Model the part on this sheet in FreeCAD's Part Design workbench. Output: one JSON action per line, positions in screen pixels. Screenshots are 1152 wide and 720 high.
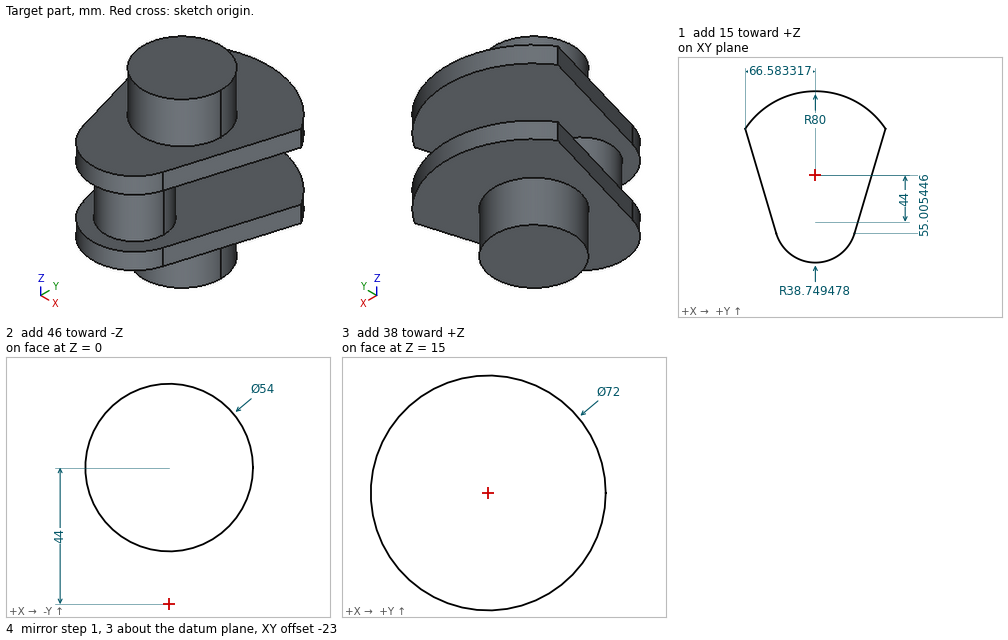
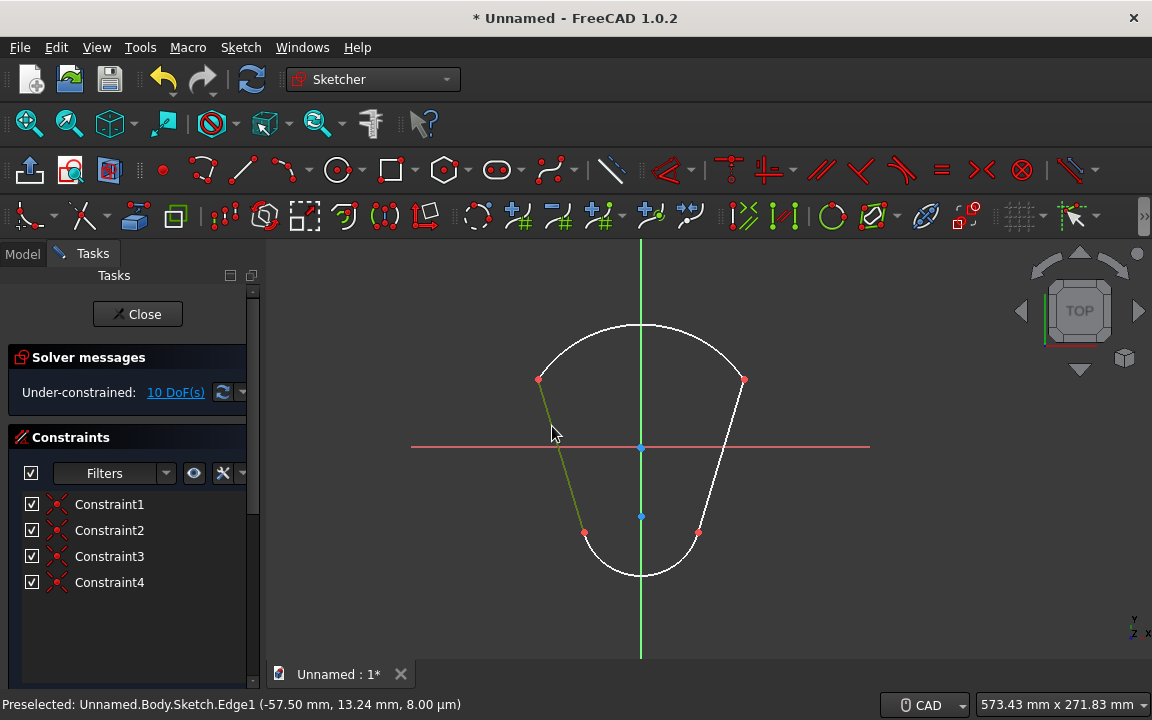
{"action": "left_click", "coordinate": [612, 568]}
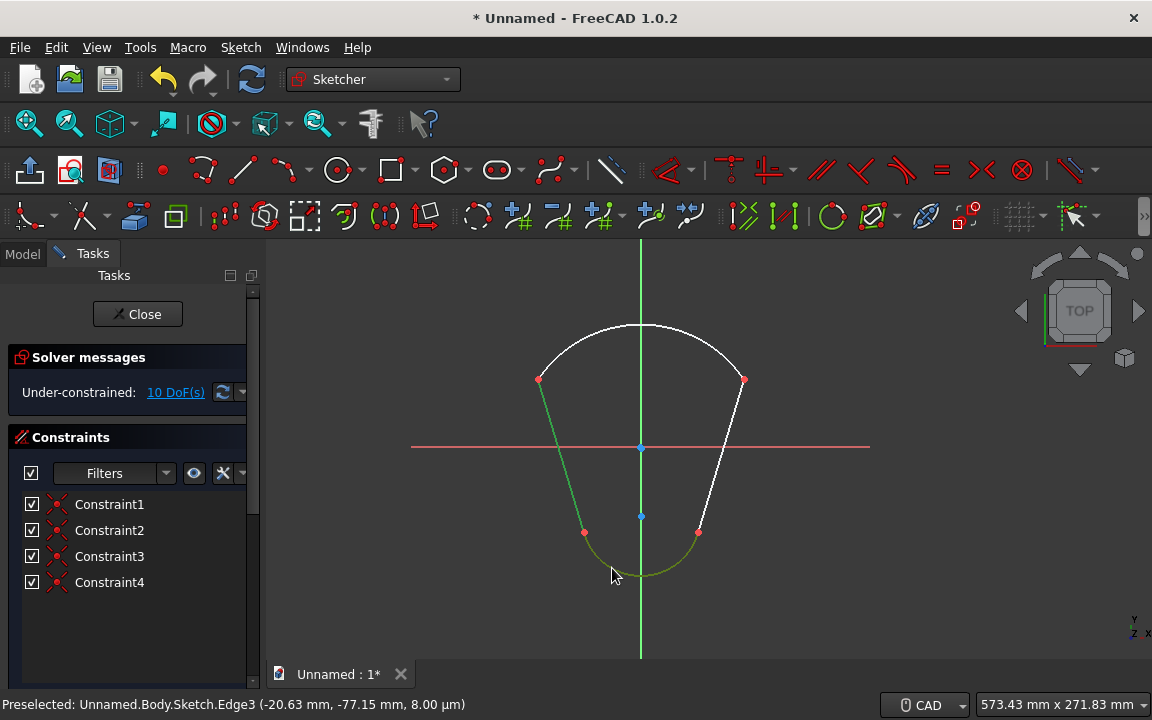
{"action": "key", "text": "t"}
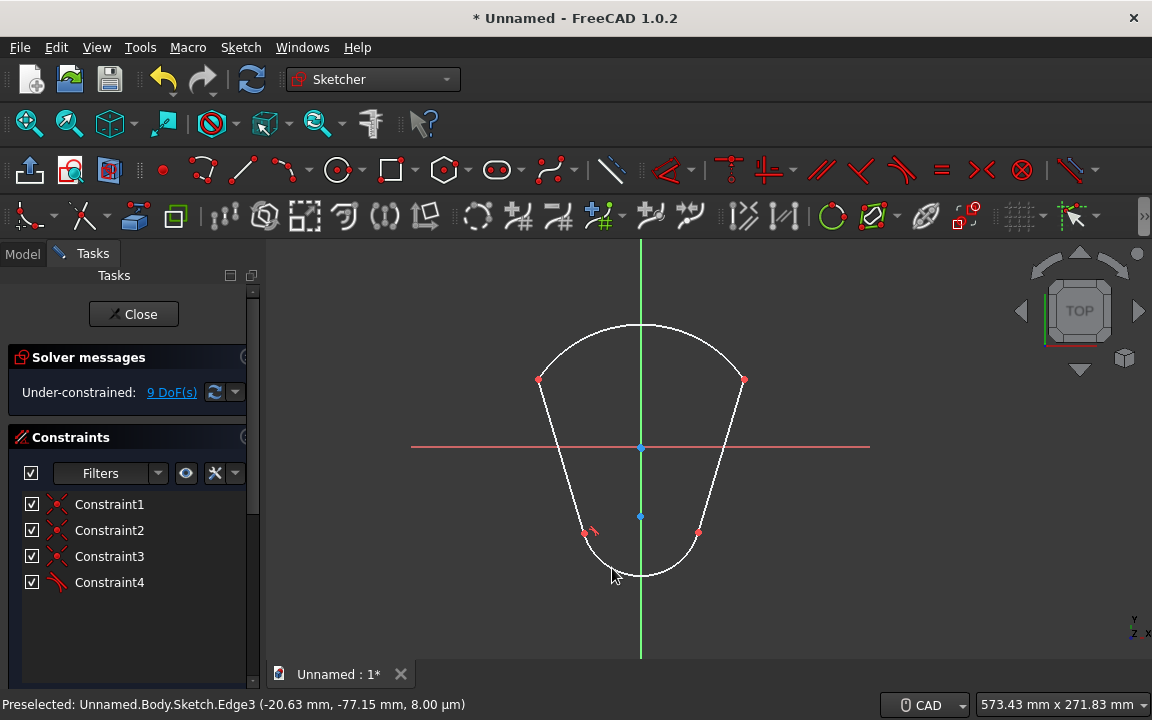
{"action": "left_click", "coordinate": [712, 487]}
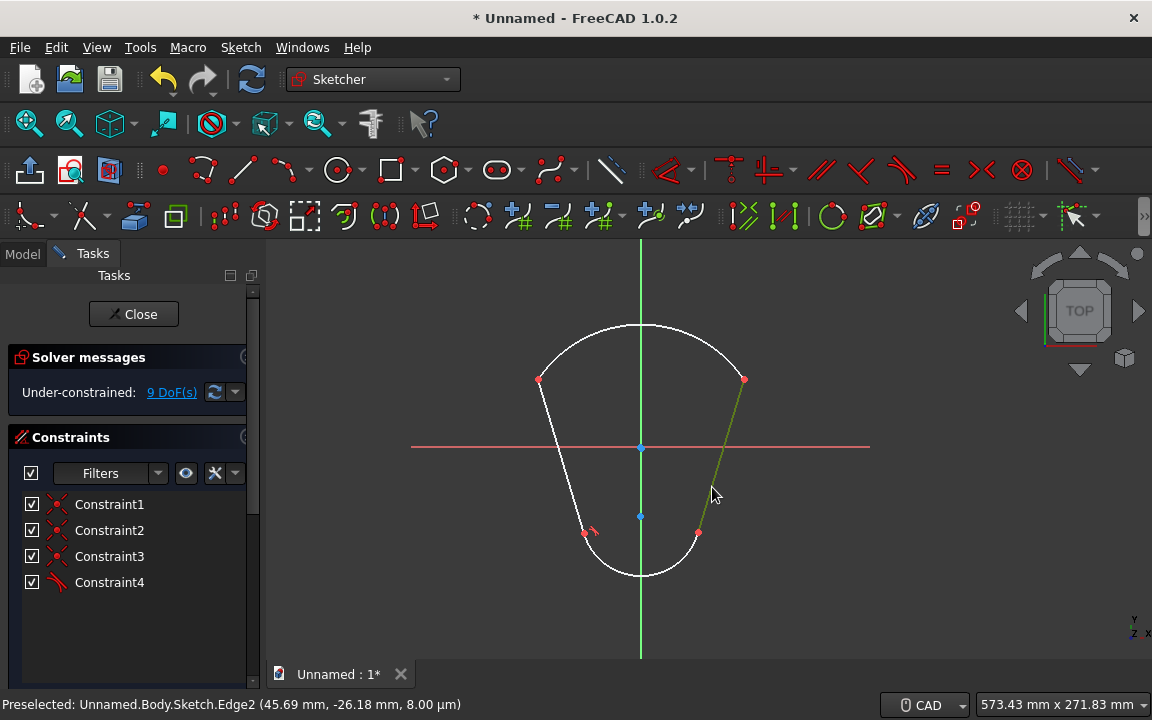
{"action": "left_click", "coordinate": [612, 569]}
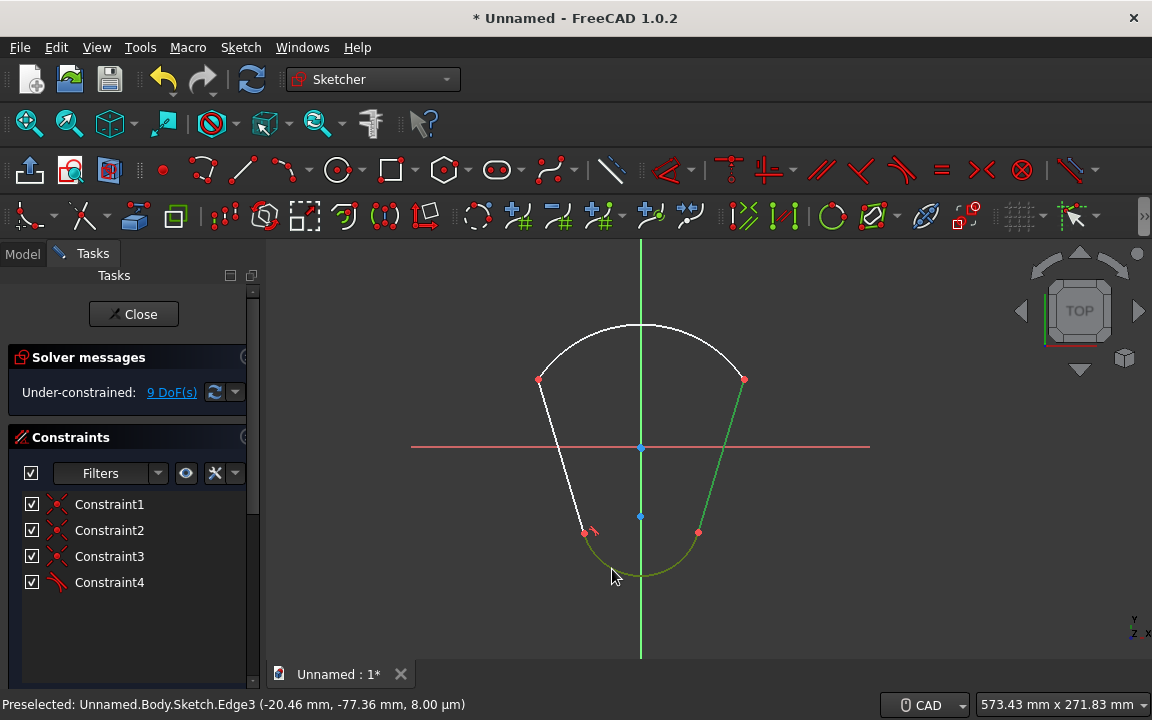
{"action": "left_click", "coordinate": [902, 170]}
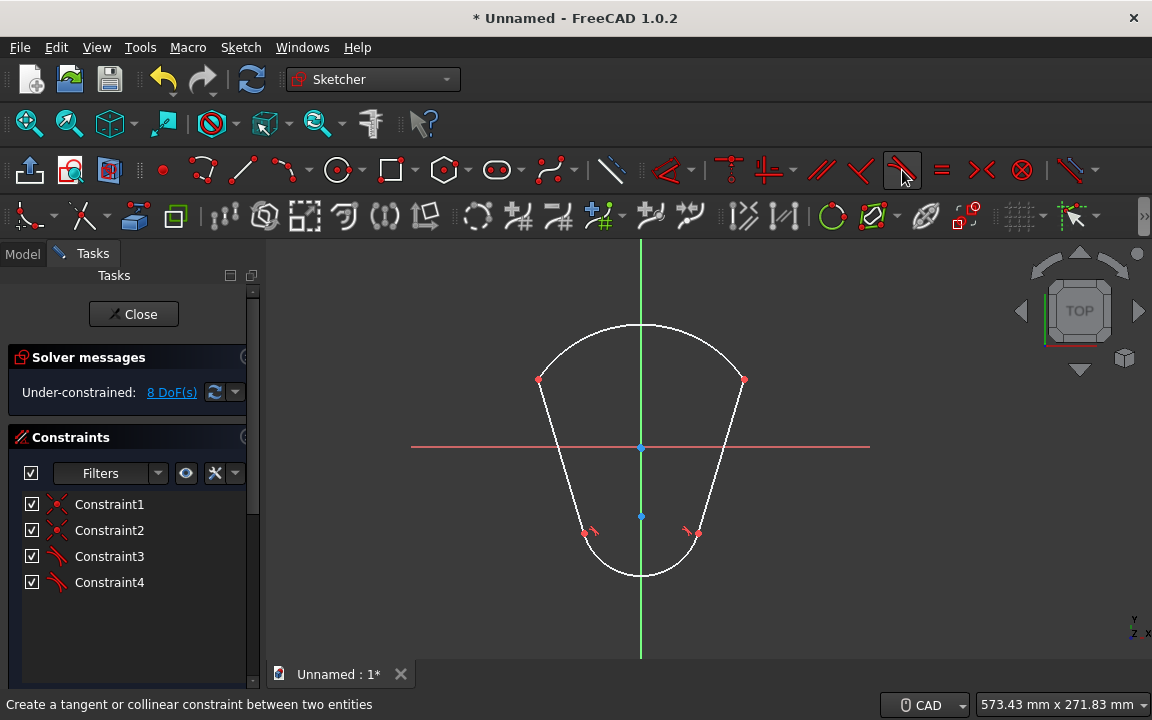
{"action": "left_click_drag", "start_coordinate": [631, 437], "coordinate": [651, 458]}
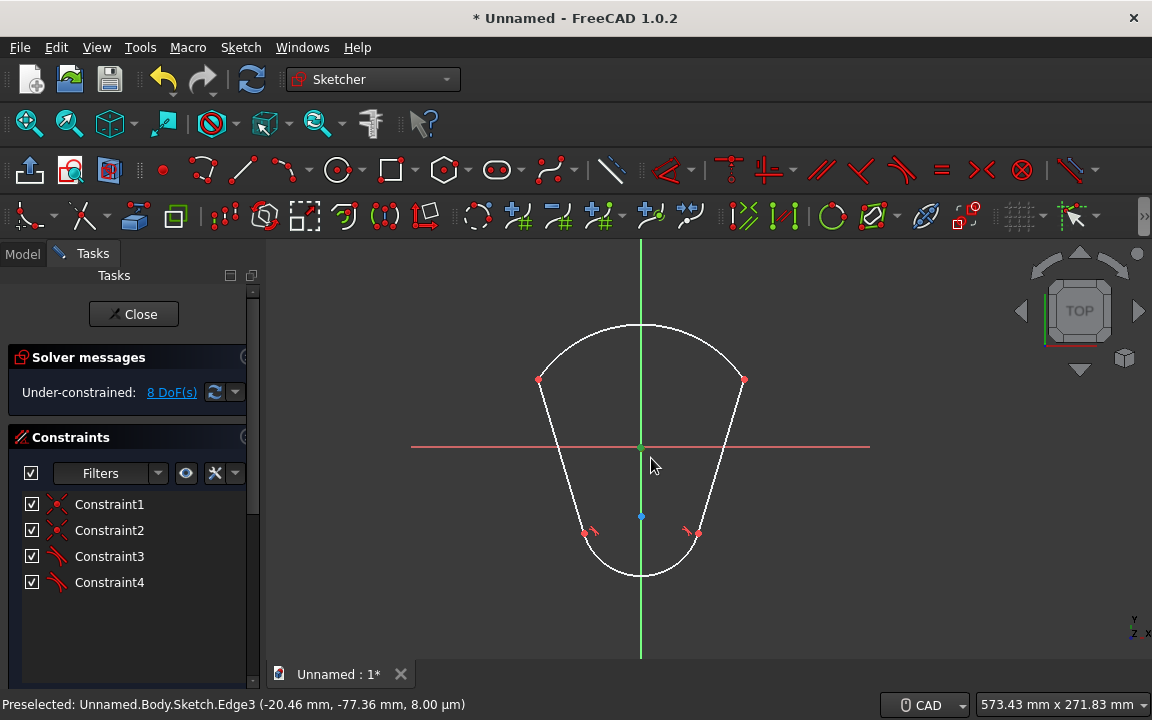
{"action": "left_click", "coordinate": [730, 170]}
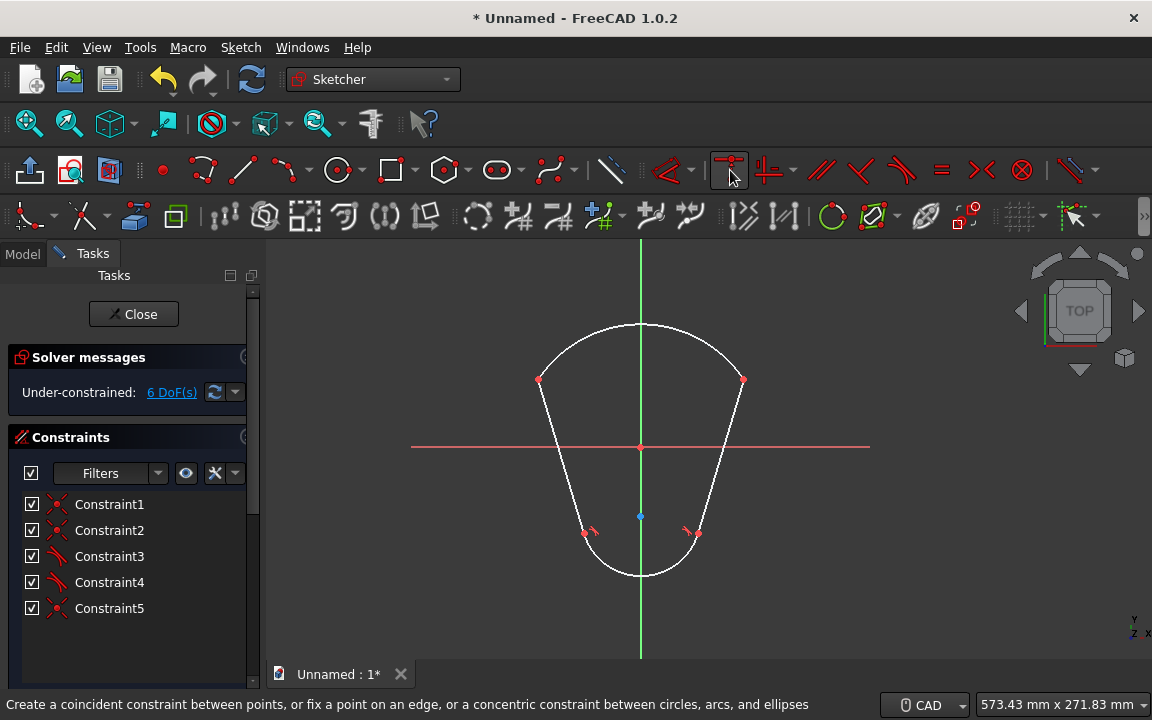
{"action": "left_click", "coordinate": [641, 517]}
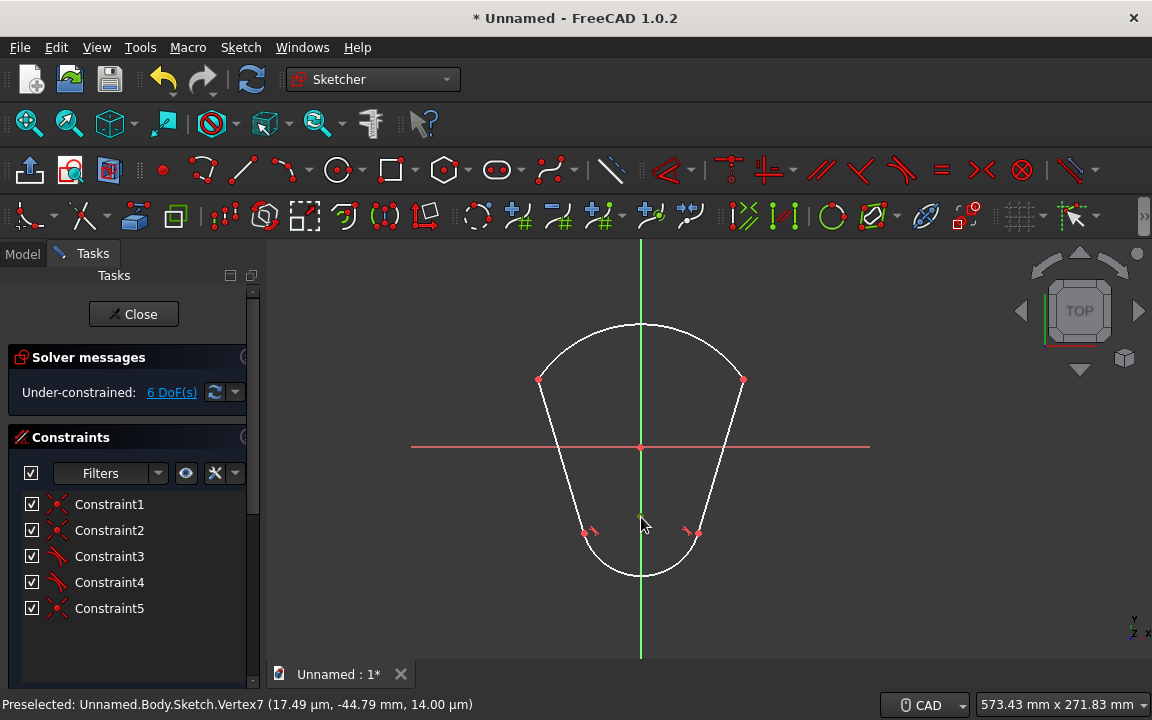
{"action": "left_click", "coordinate": [641, 527]}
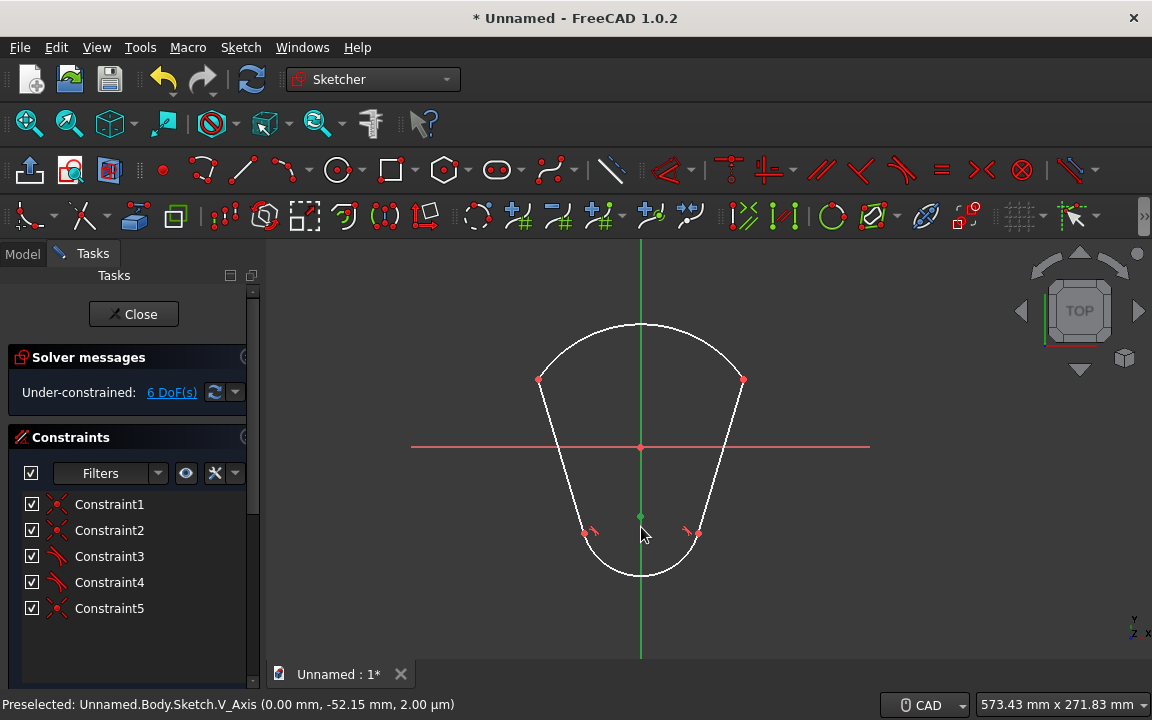
{"action": "left_click", "coordinate": [730, 170]}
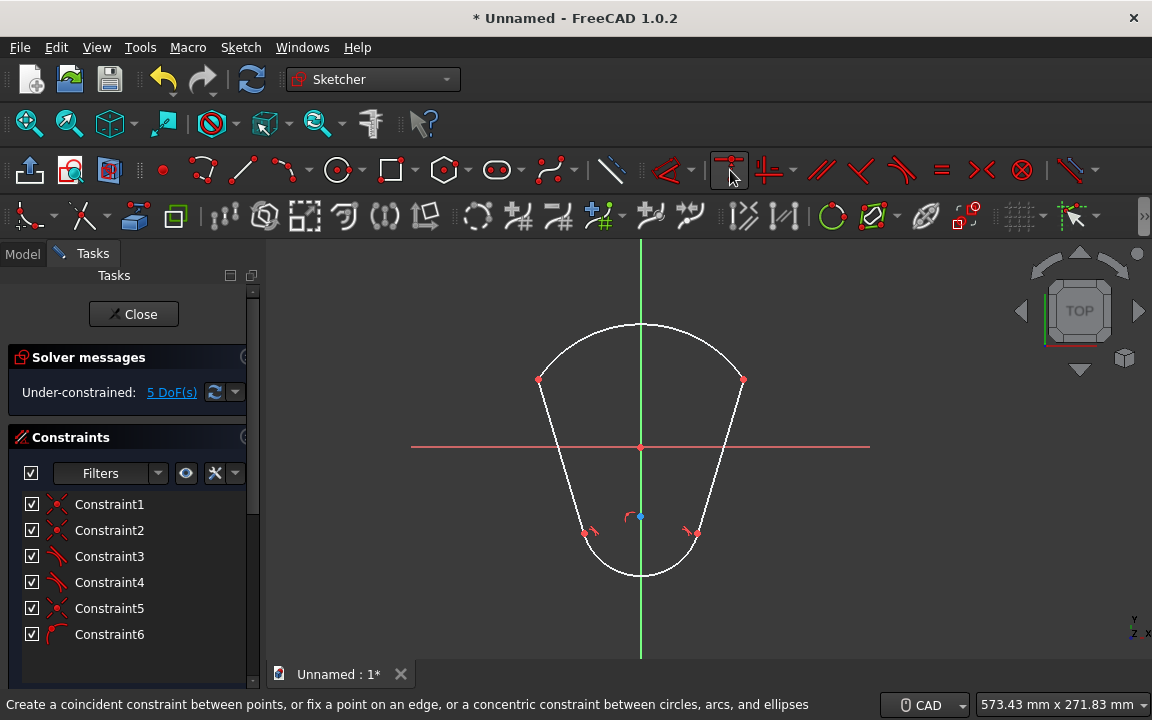
{"action": "left_click", "coordinate": [666, 170]}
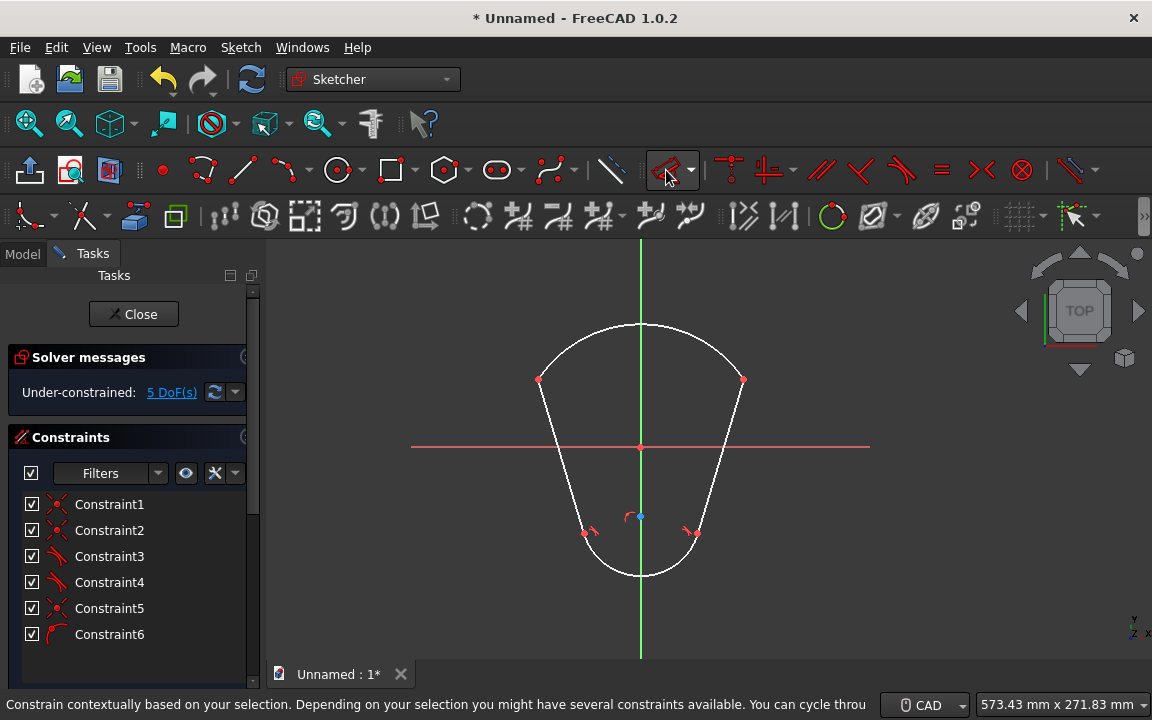
{"action": "left_click", "coordinate": [612, 568]}
{"action": "left_click", "coordinate": [596, 596]}